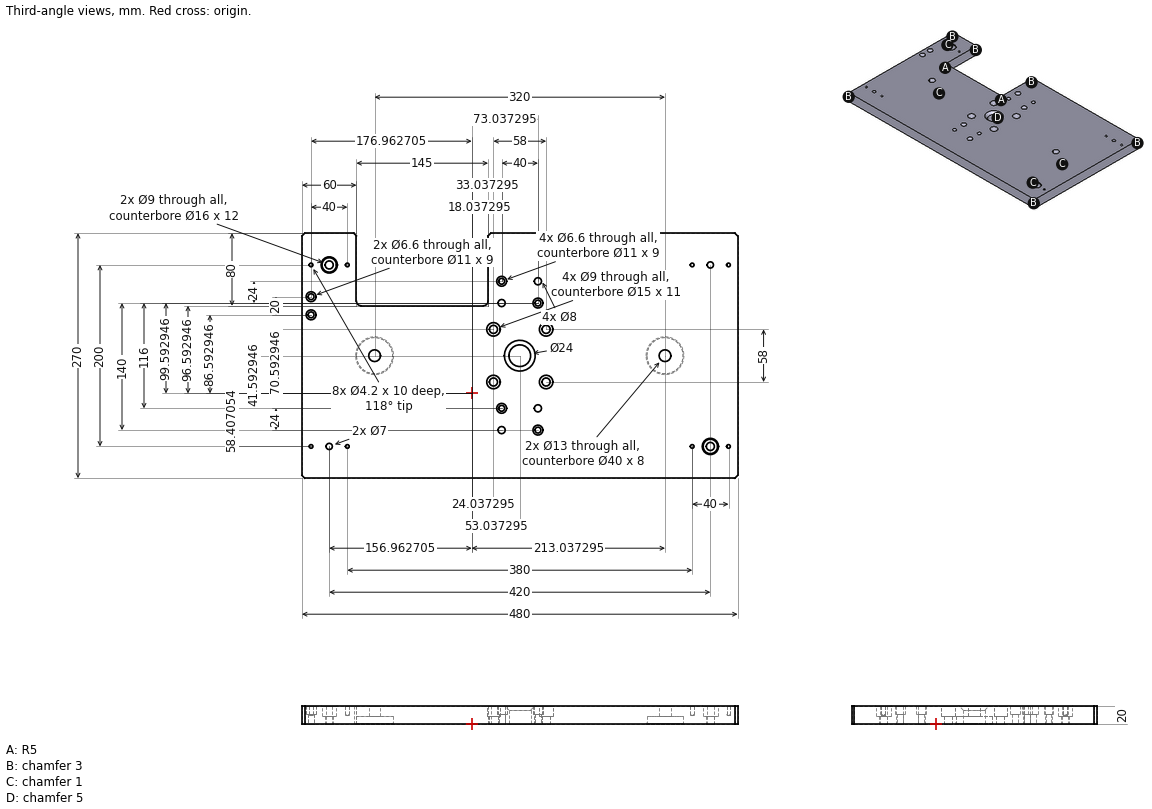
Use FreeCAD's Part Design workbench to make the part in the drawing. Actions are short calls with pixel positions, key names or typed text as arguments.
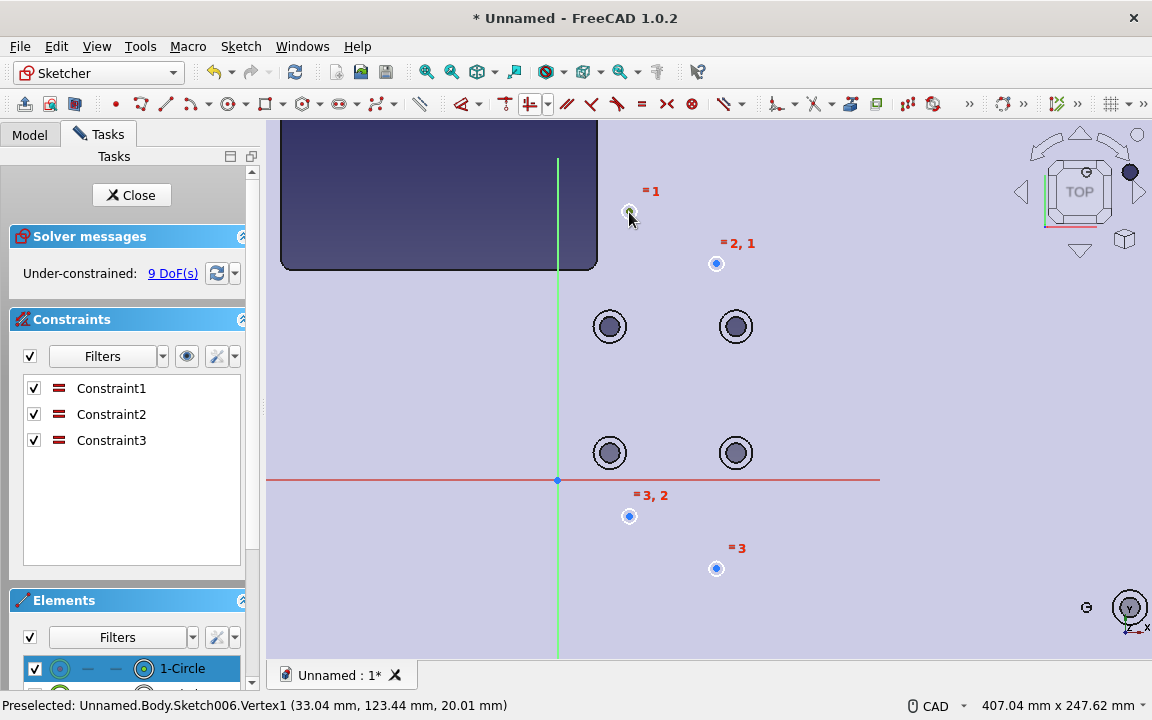
click(629, 516)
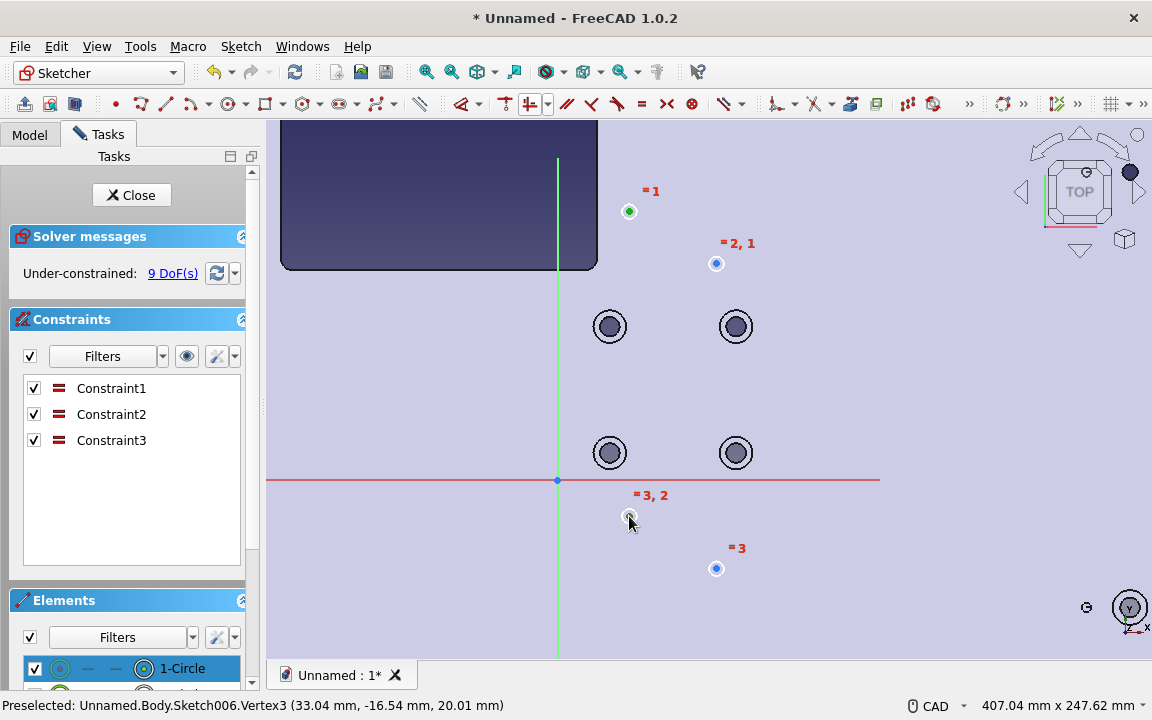
key(v)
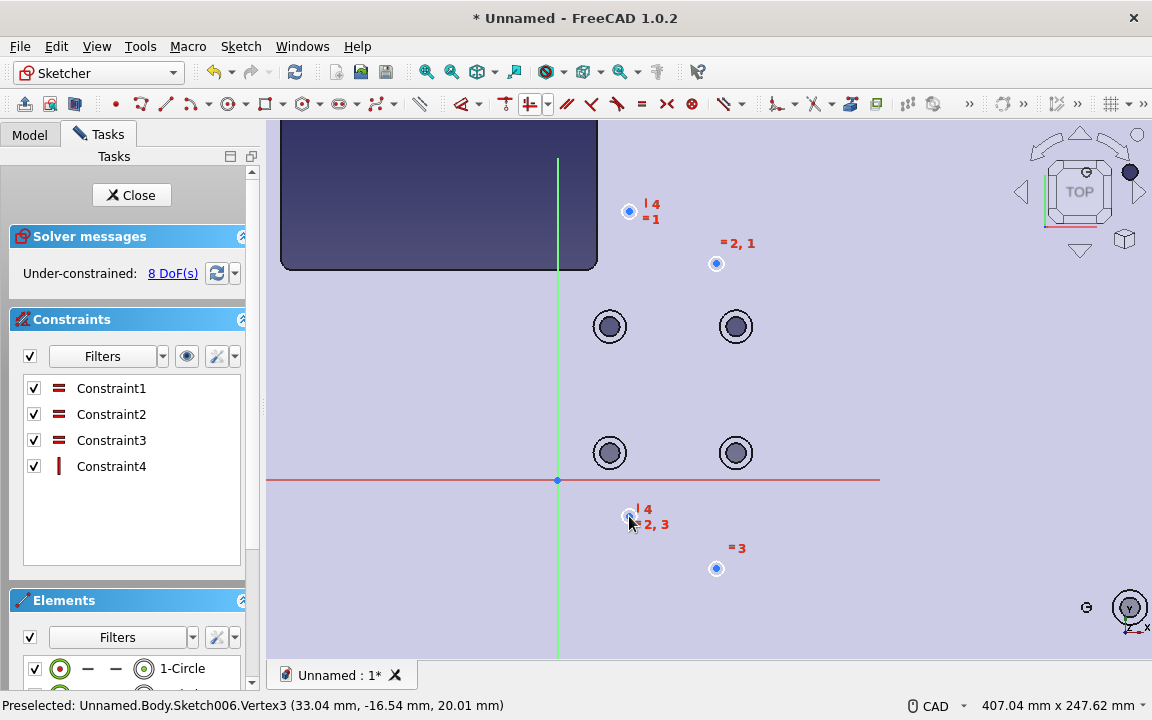
click(716, 264)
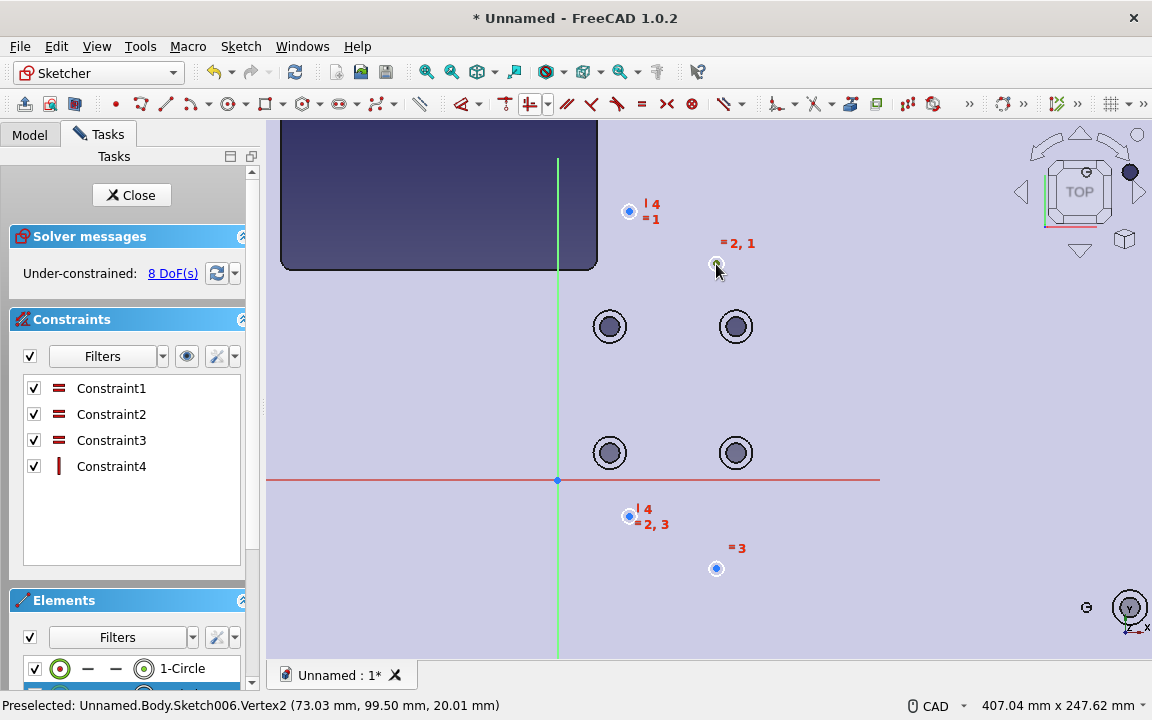
click(717, 569)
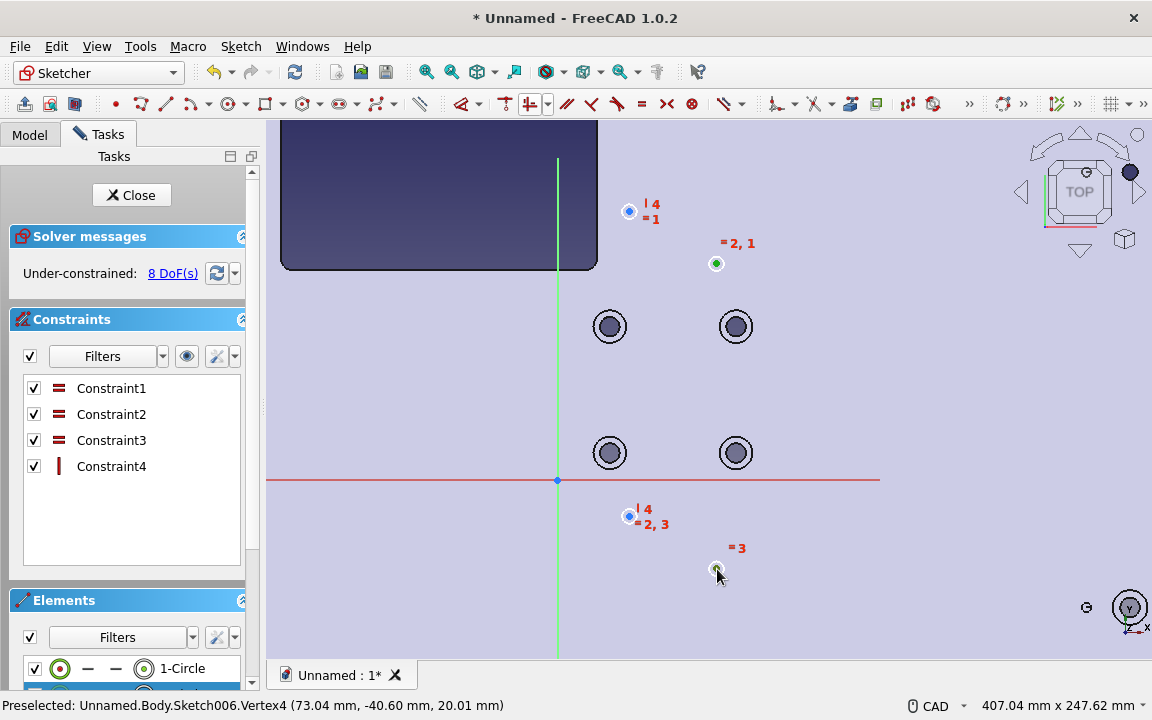
click(548, 104)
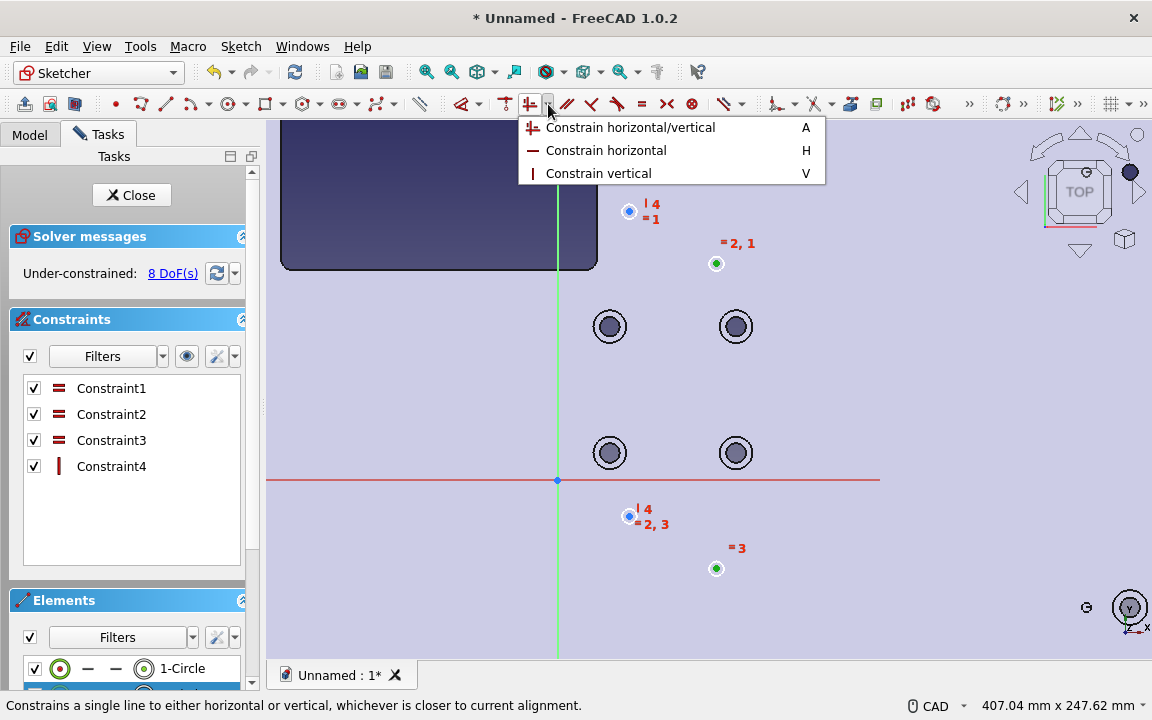
click(672, 174)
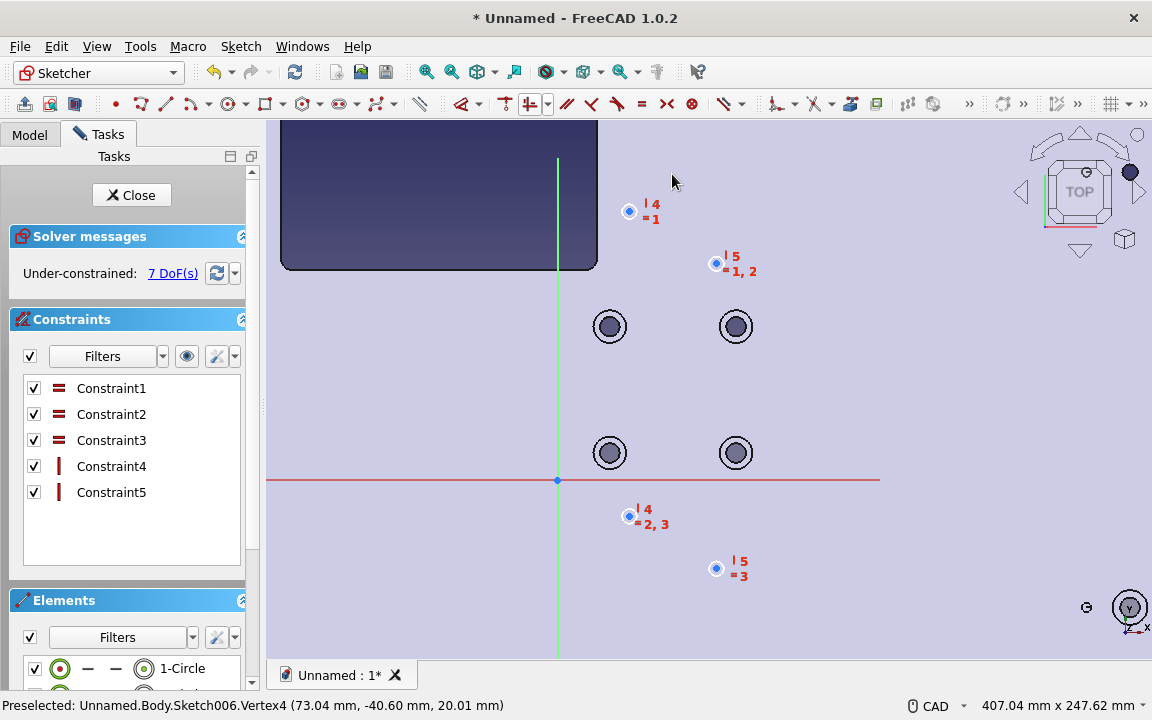
key(d)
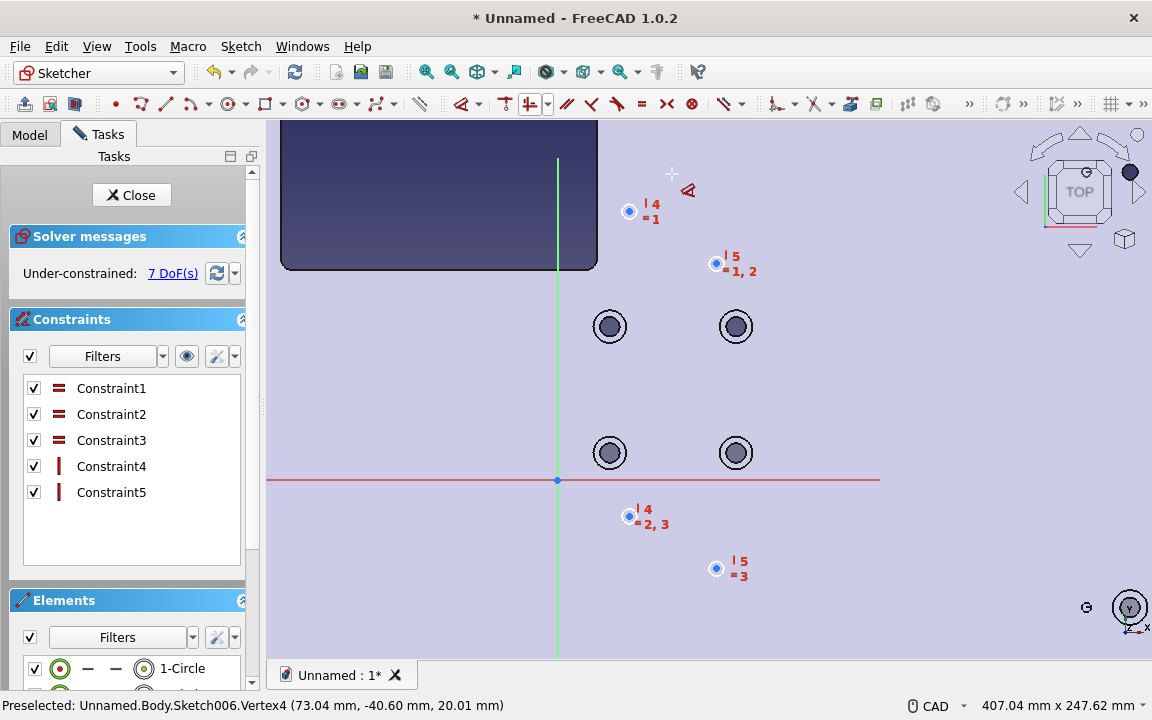
scroll(635, 207, up, 6)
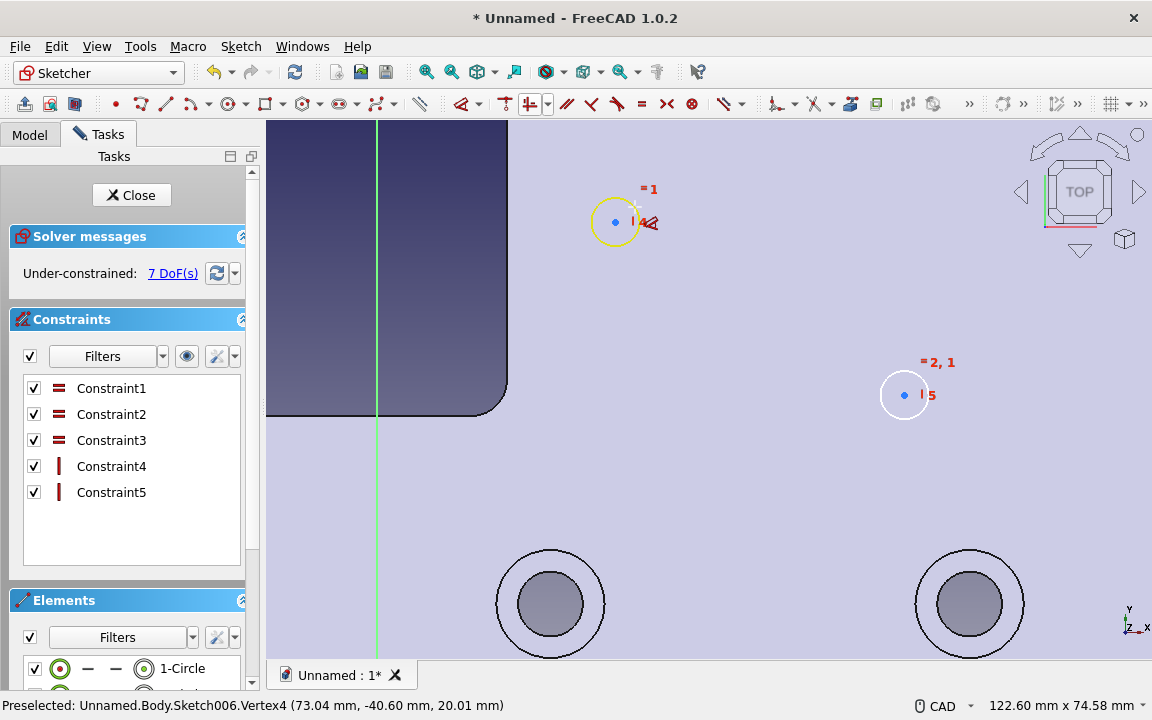
click(633, 205)
click(656, 183)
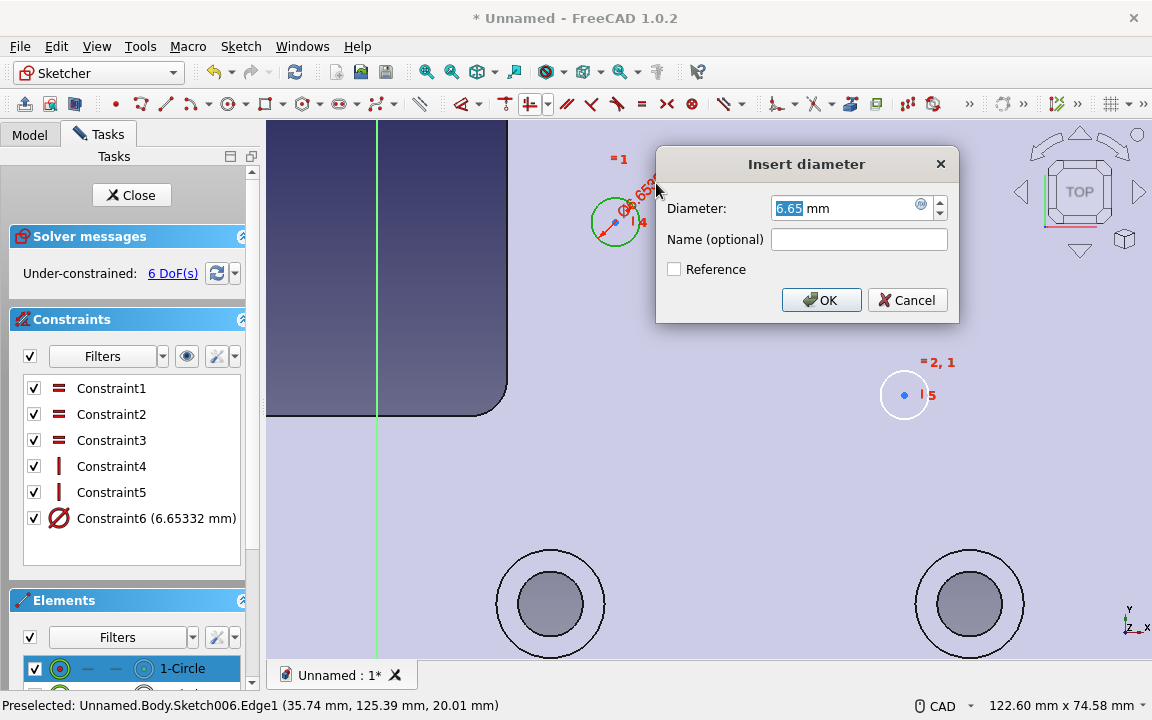
text(6.6)
key(Return)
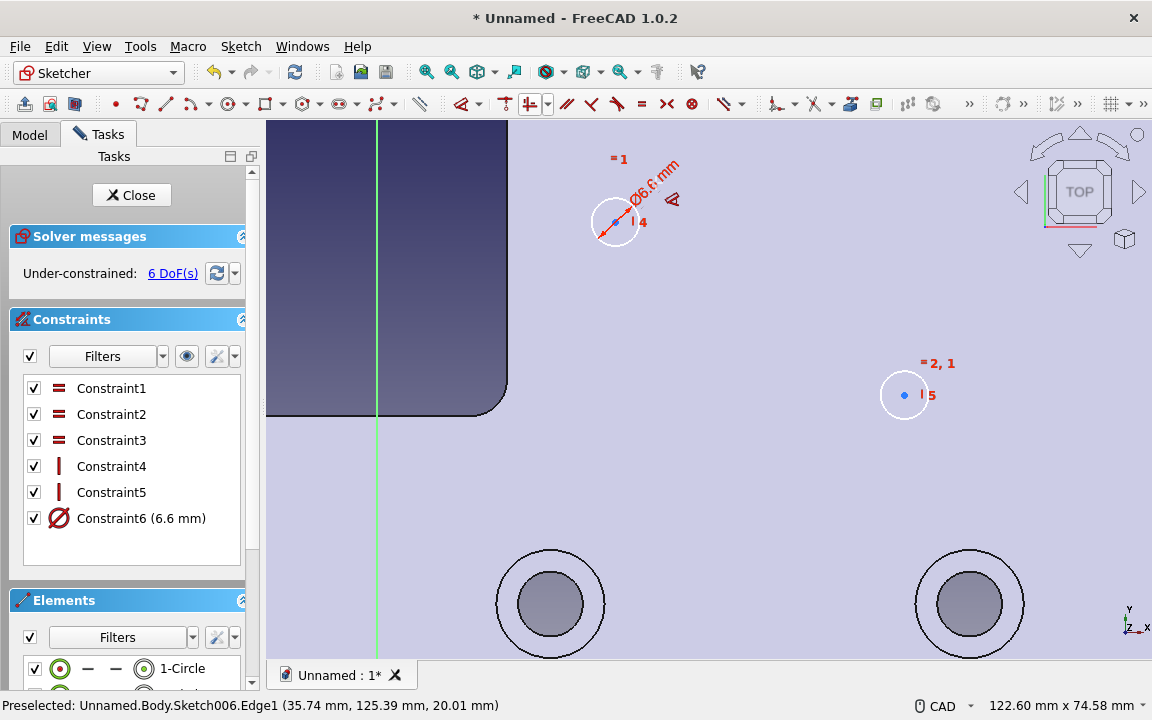
click(616, 222)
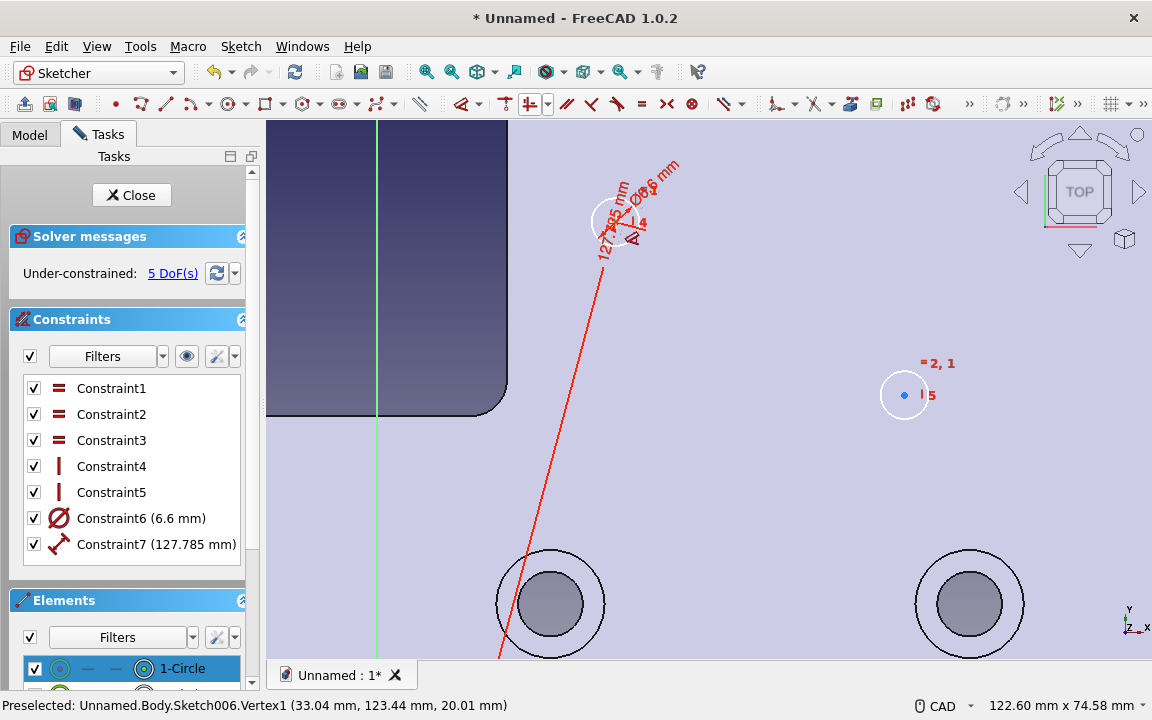
click(905, 395)
click(760, 188)